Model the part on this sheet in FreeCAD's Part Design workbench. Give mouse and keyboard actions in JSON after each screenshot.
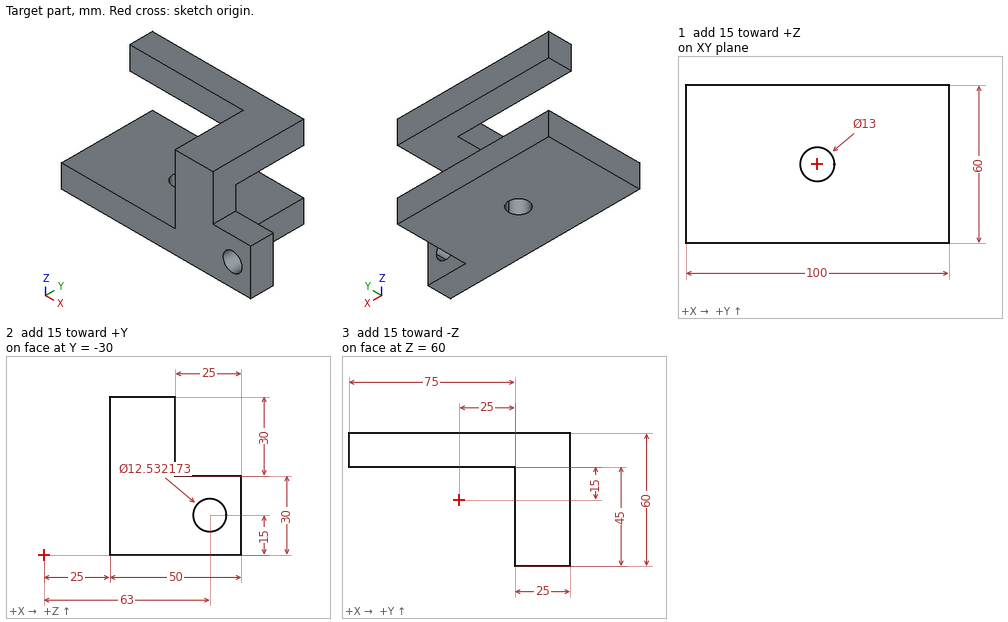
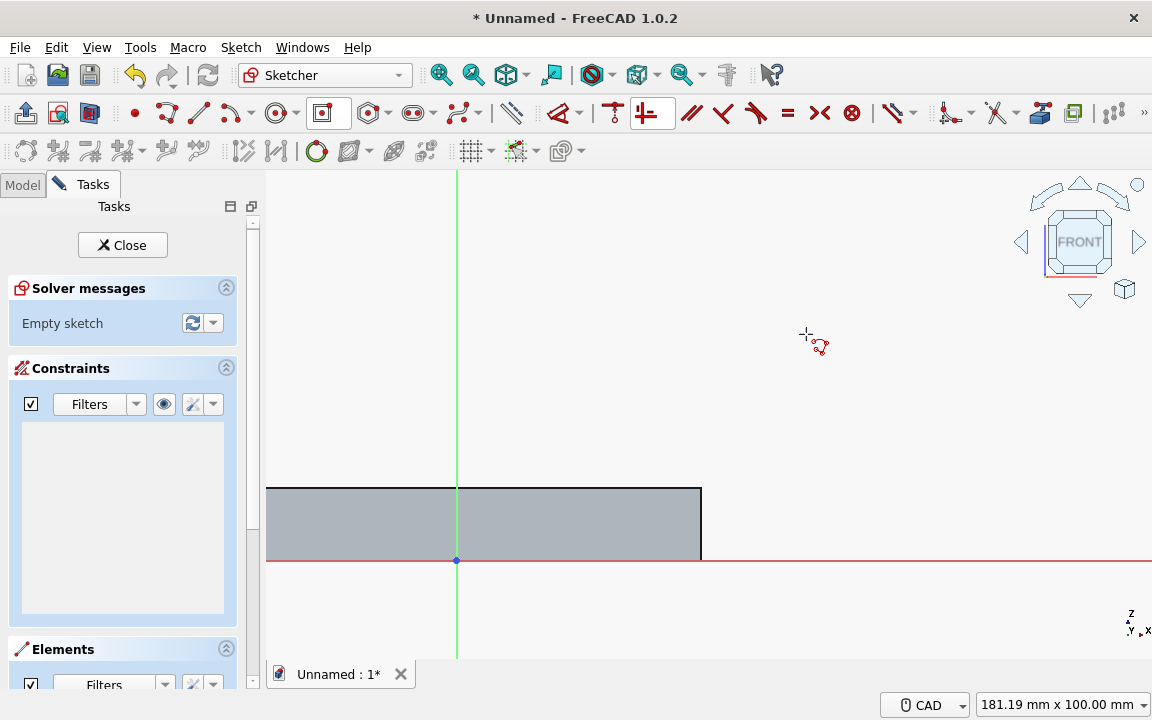
{"action": "left_click", "coordinate": [579, 561]}
{"action": "left_click", "coordinate": [824, 552]}
{"action": "left_click", "coordinate": [824, 414]}
{"action": "left_click", "coordinate": [701, 414]}
{"action": "left_click", "coordinate": [701, 267]}
{"action": "left_click", "coordinate": [579, 267]}
{"action": "left_click", "coordinate": [579, 561]}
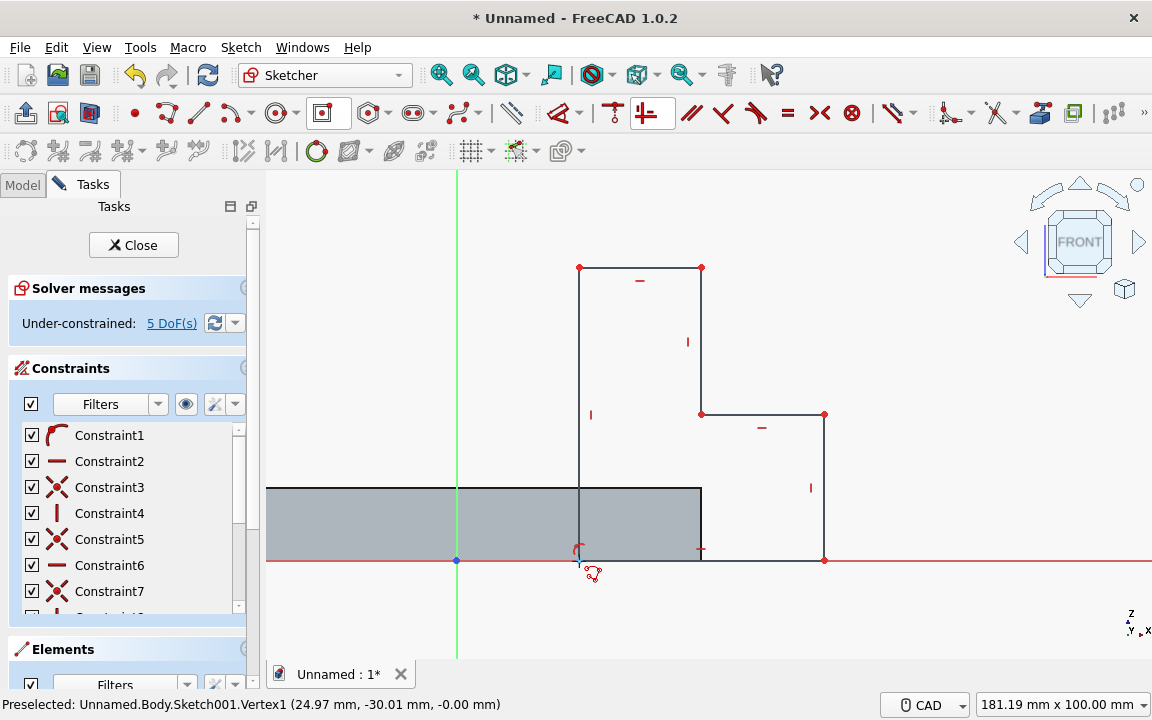
{"action": "left_click", "coordinate": [276, 114]}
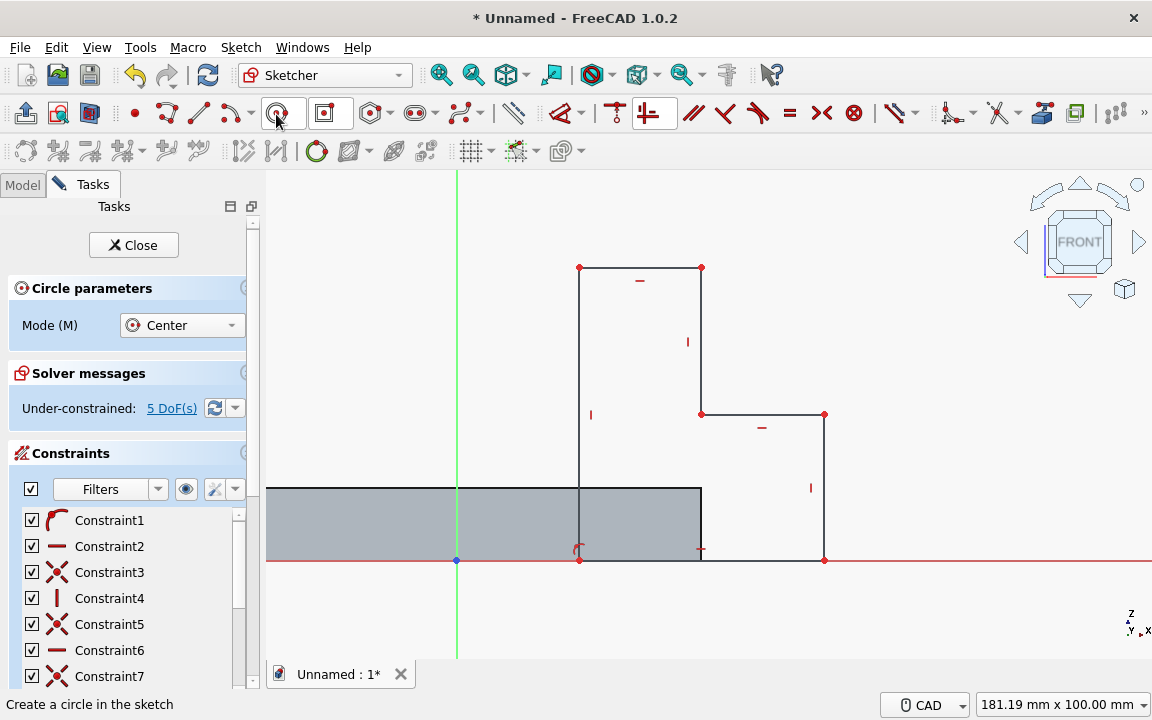
{"action": "left_click", "coordinate": [765, 488]}
{"action": "left_click", "coordinate": [787, 466]}
{"action": "key", "text": "Escape"}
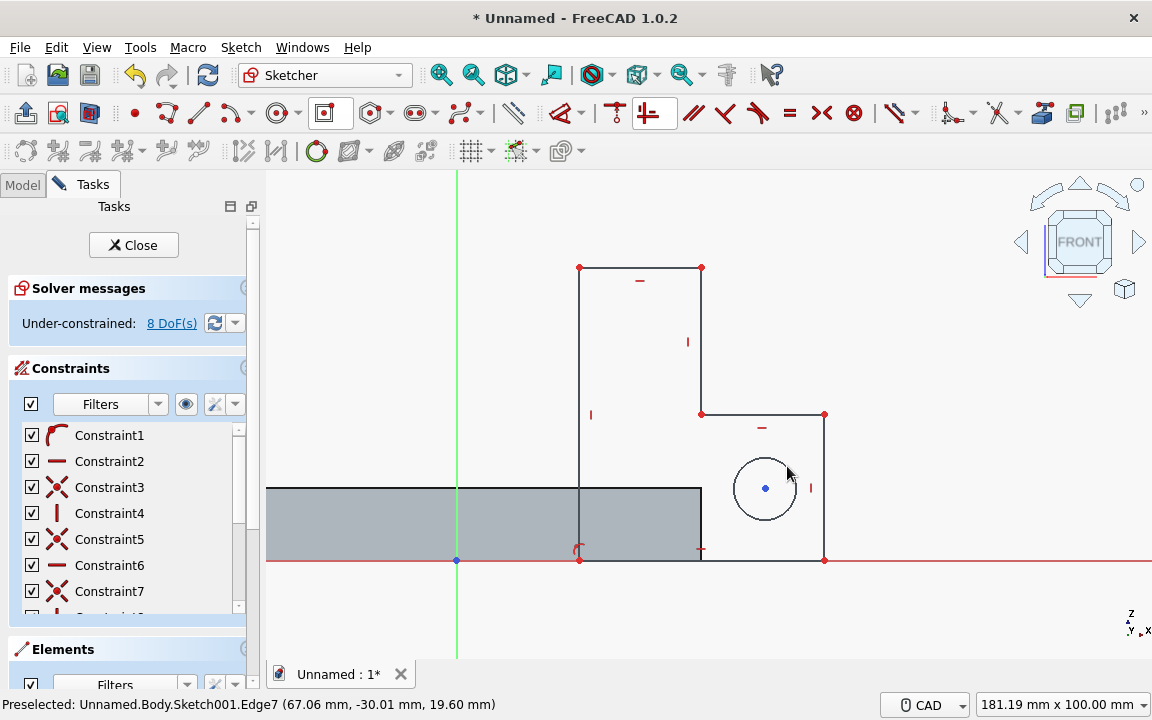
{"action": "left_click", "coordinate": [560, 114]}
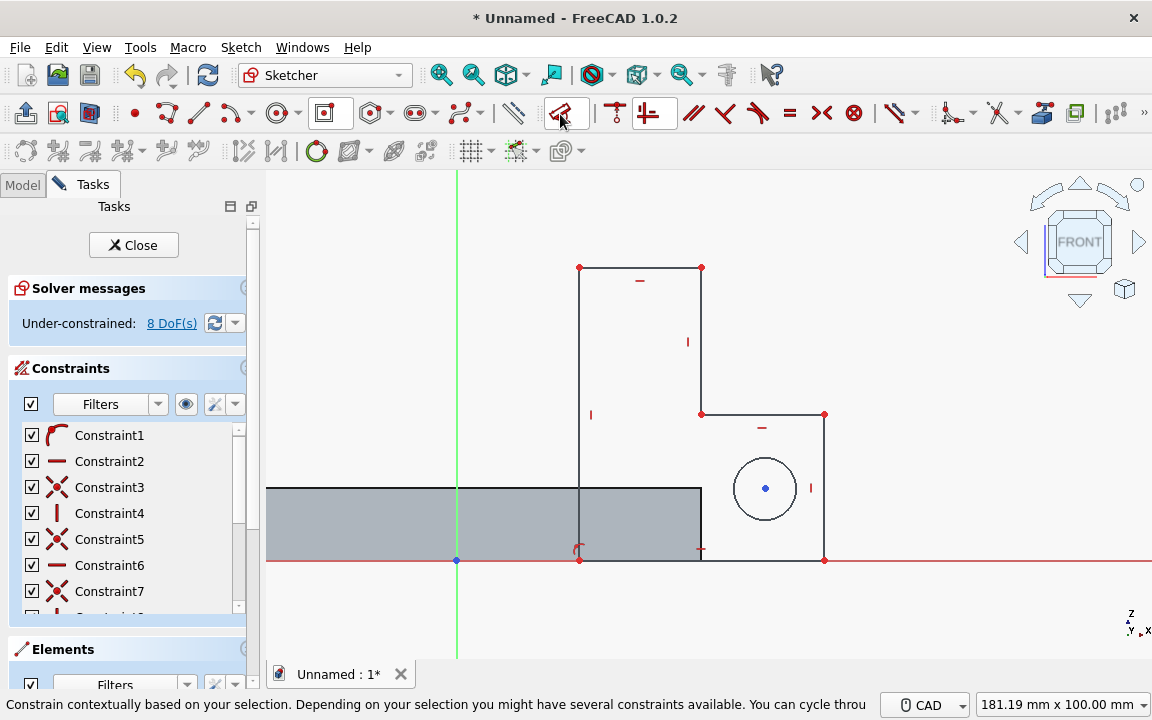
{"action": "left_click", "coordinate": [787, 467]}
{"action": "left_click", "coordinate": [810, 444]}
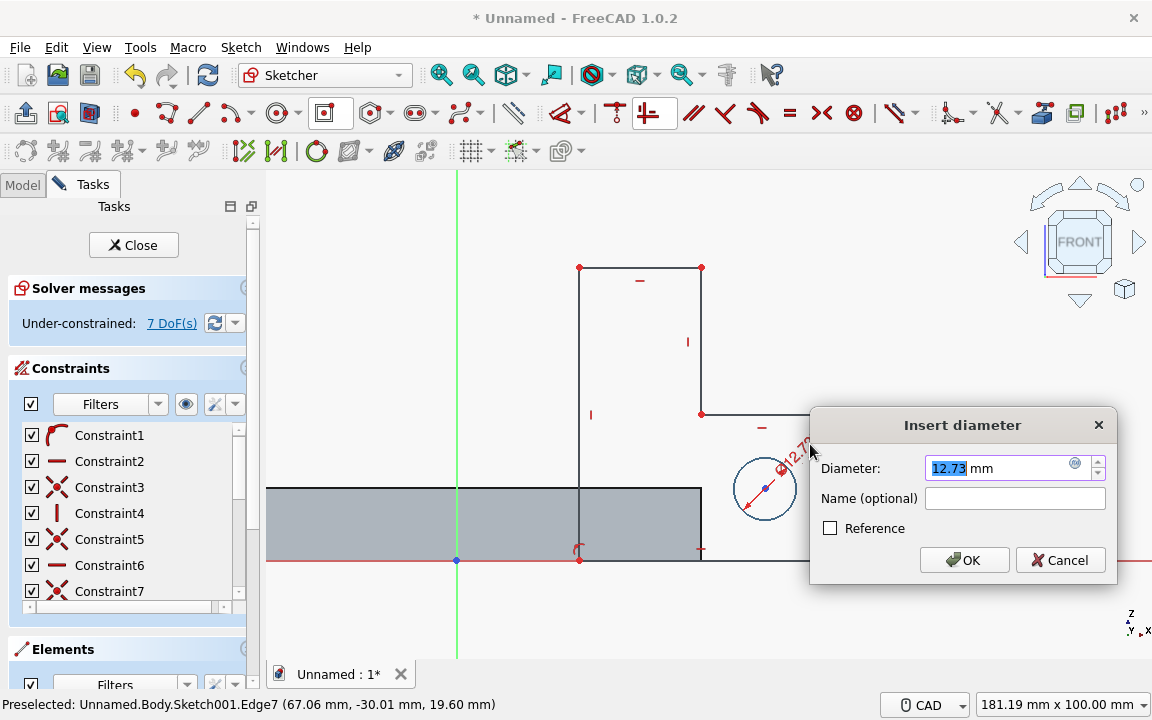
{"action": "type", "text": "12.532173"}
{"action": "key", "text": "Return"}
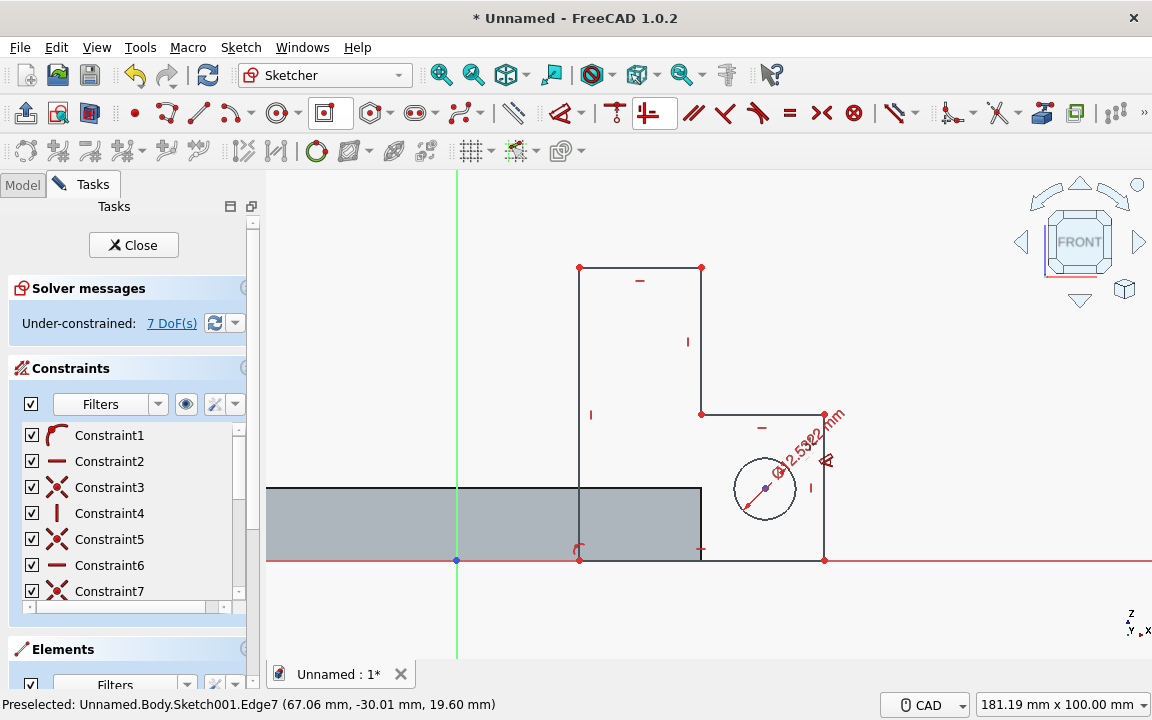
{"action": "left_click", "coordinate": [652, 561]}
{"action": "left_click", "coordinate": [702, 595]}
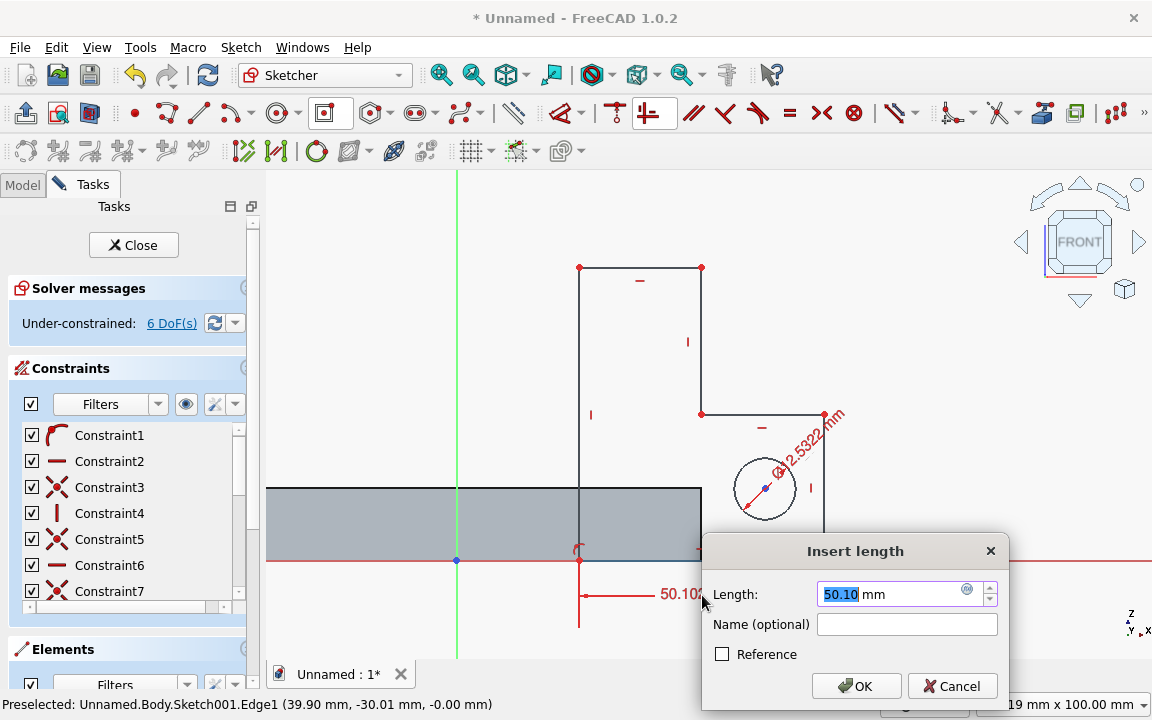
{"action": "type", "text": "50"}
{"action": "key", "text": "Return"}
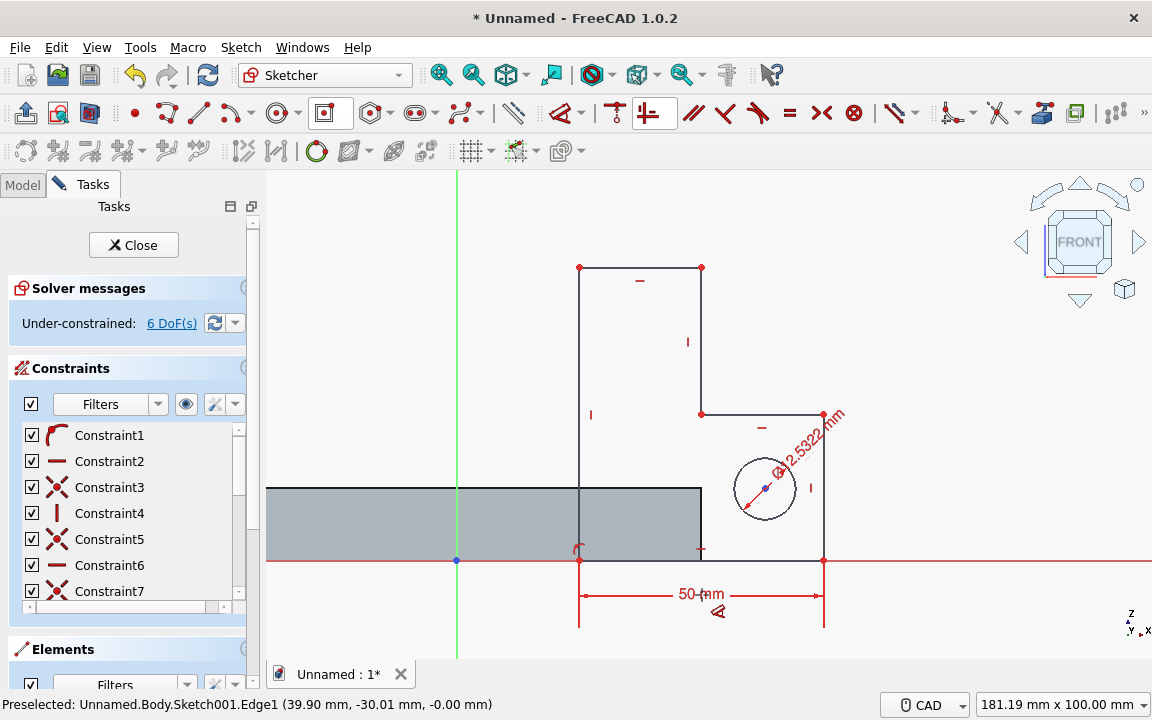
{"action": "left_click", "coordinate": [824, 517]}
{"action": "left_click", "coordinate": [858, 488]}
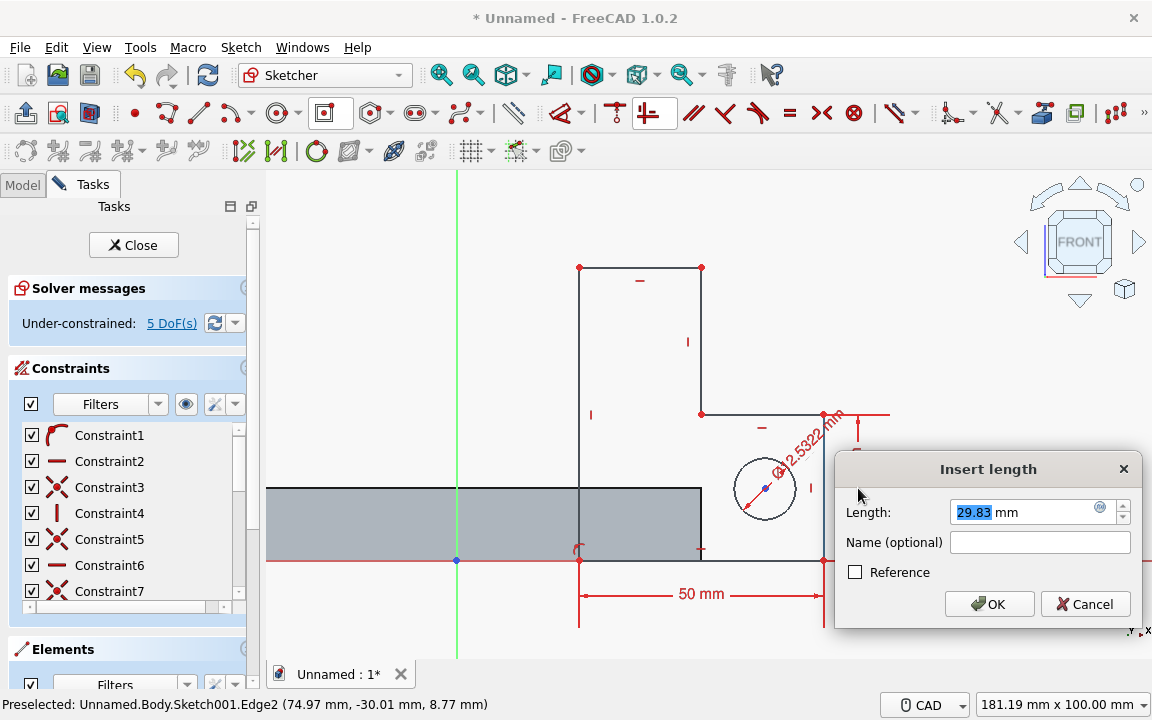
{"action": "type", "text": "30"}
{"action": "key", "text": "Return"}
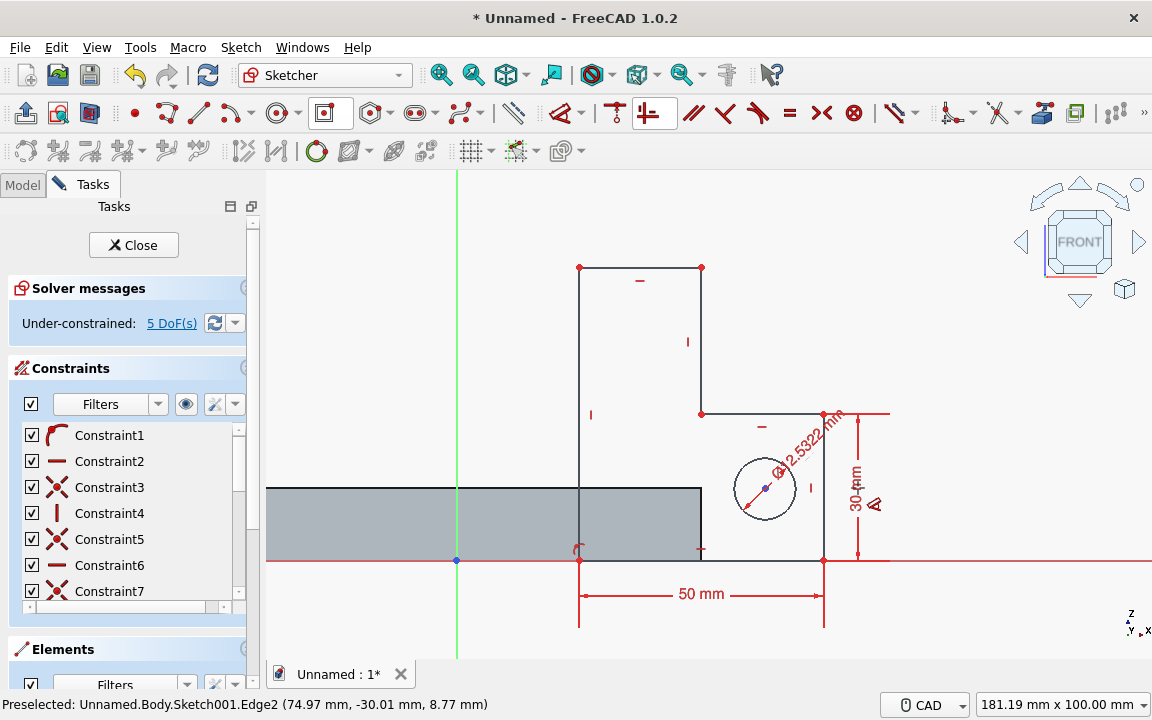
{"action": "left_click", "coordinate": [787, 414]}
{"action": "left_click", "coordinate": [734, 448]}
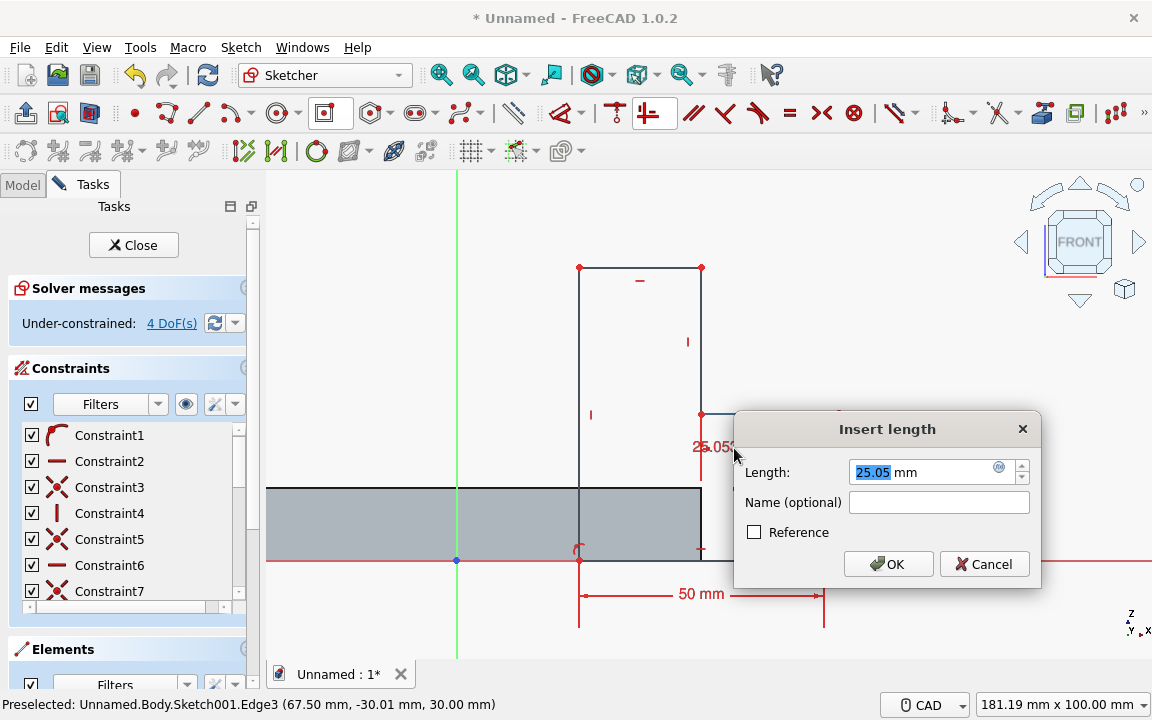
{"action": "type", "text": "25"}
{"action": "key", "text": "Return"}